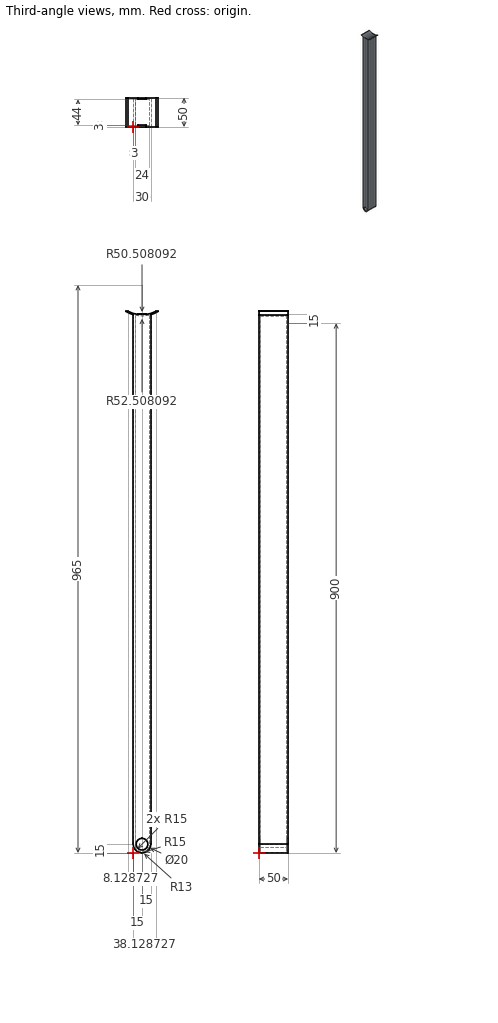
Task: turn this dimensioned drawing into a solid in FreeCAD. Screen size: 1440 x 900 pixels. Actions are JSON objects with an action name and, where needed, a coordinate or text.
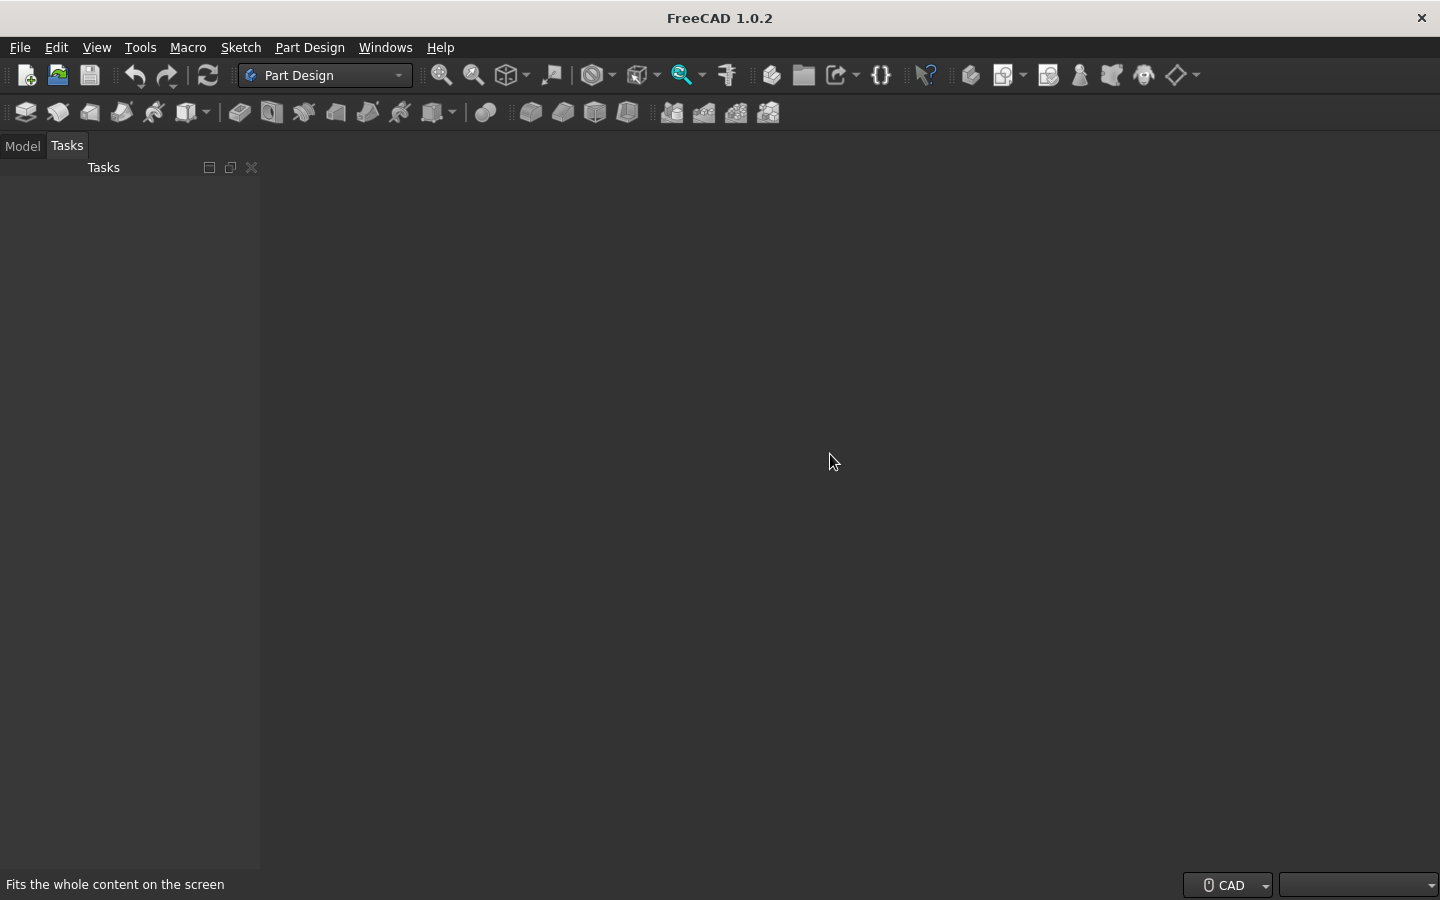
{"action": "left_click", "coordinate": [26, 76]}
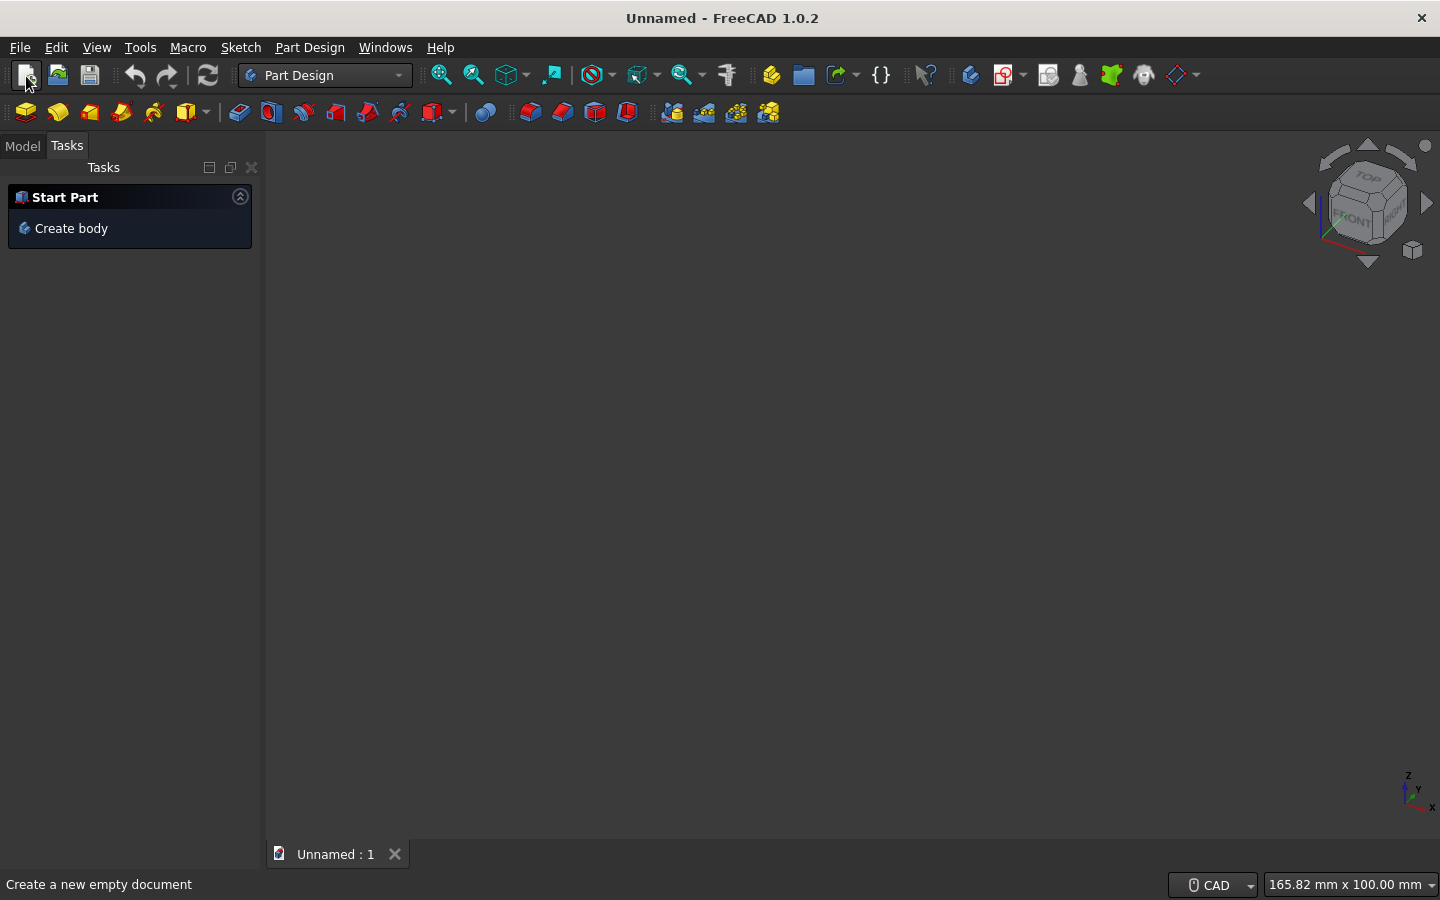
{"action": "left_click", "coordinate": [1004, 76]}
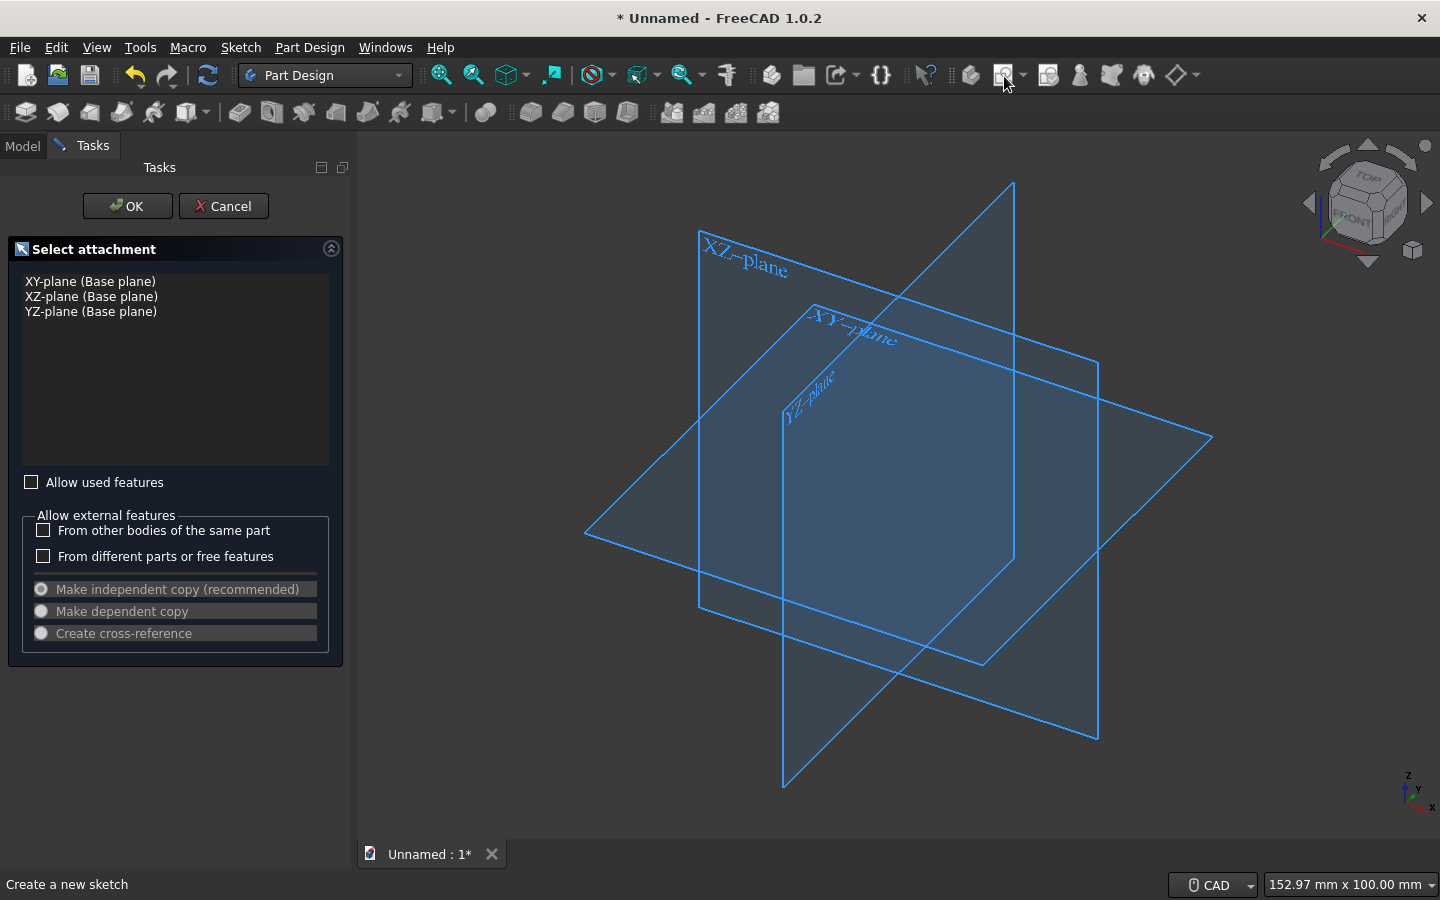
{"action": "left_click", "coordinate": [82, 282]}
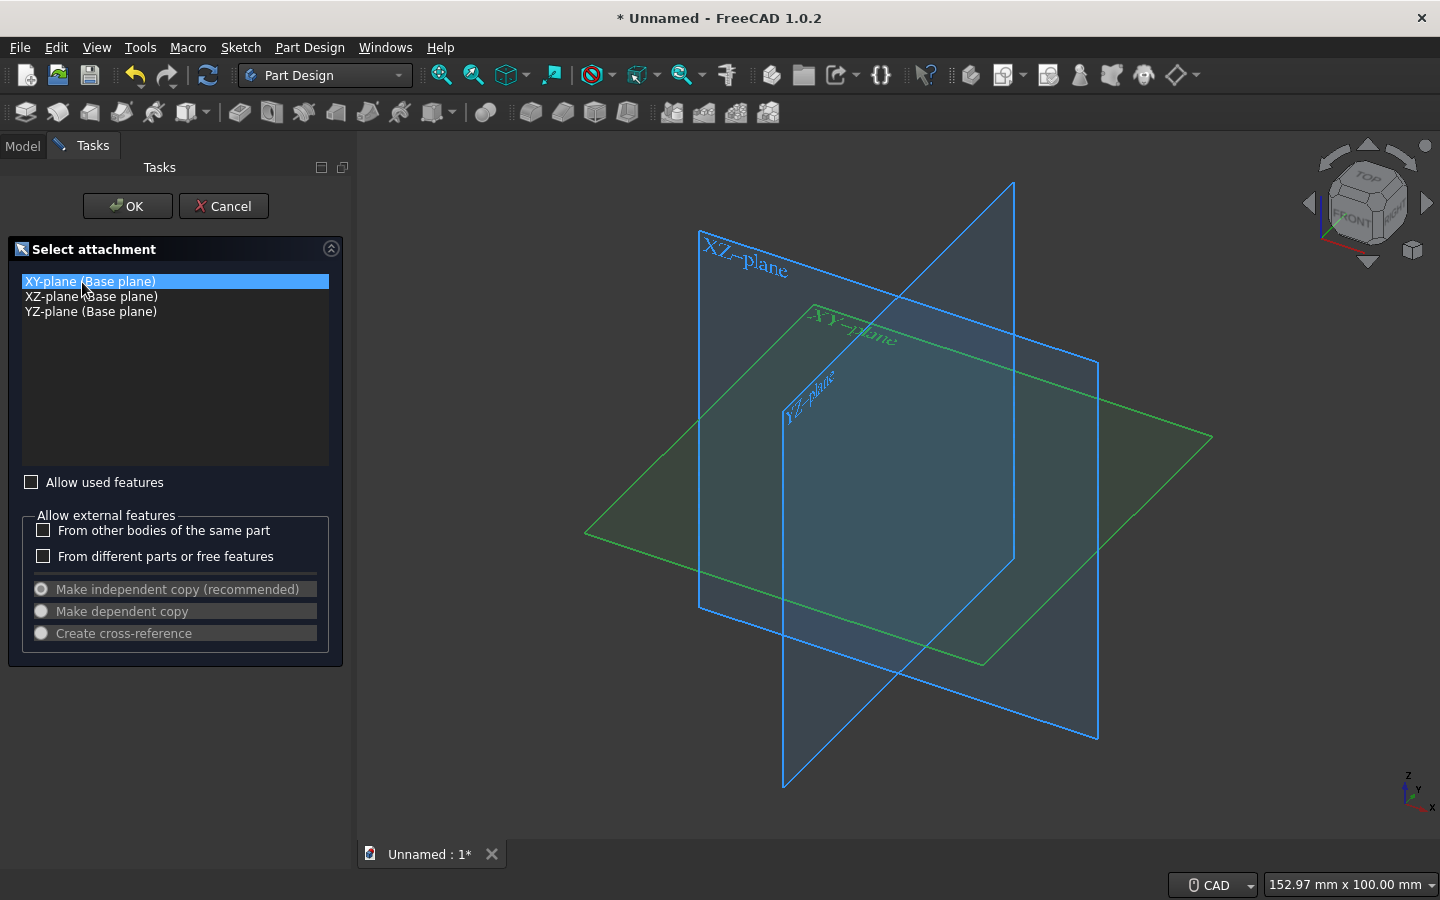
{"action": "left_click", "coordinate": [128, 206]}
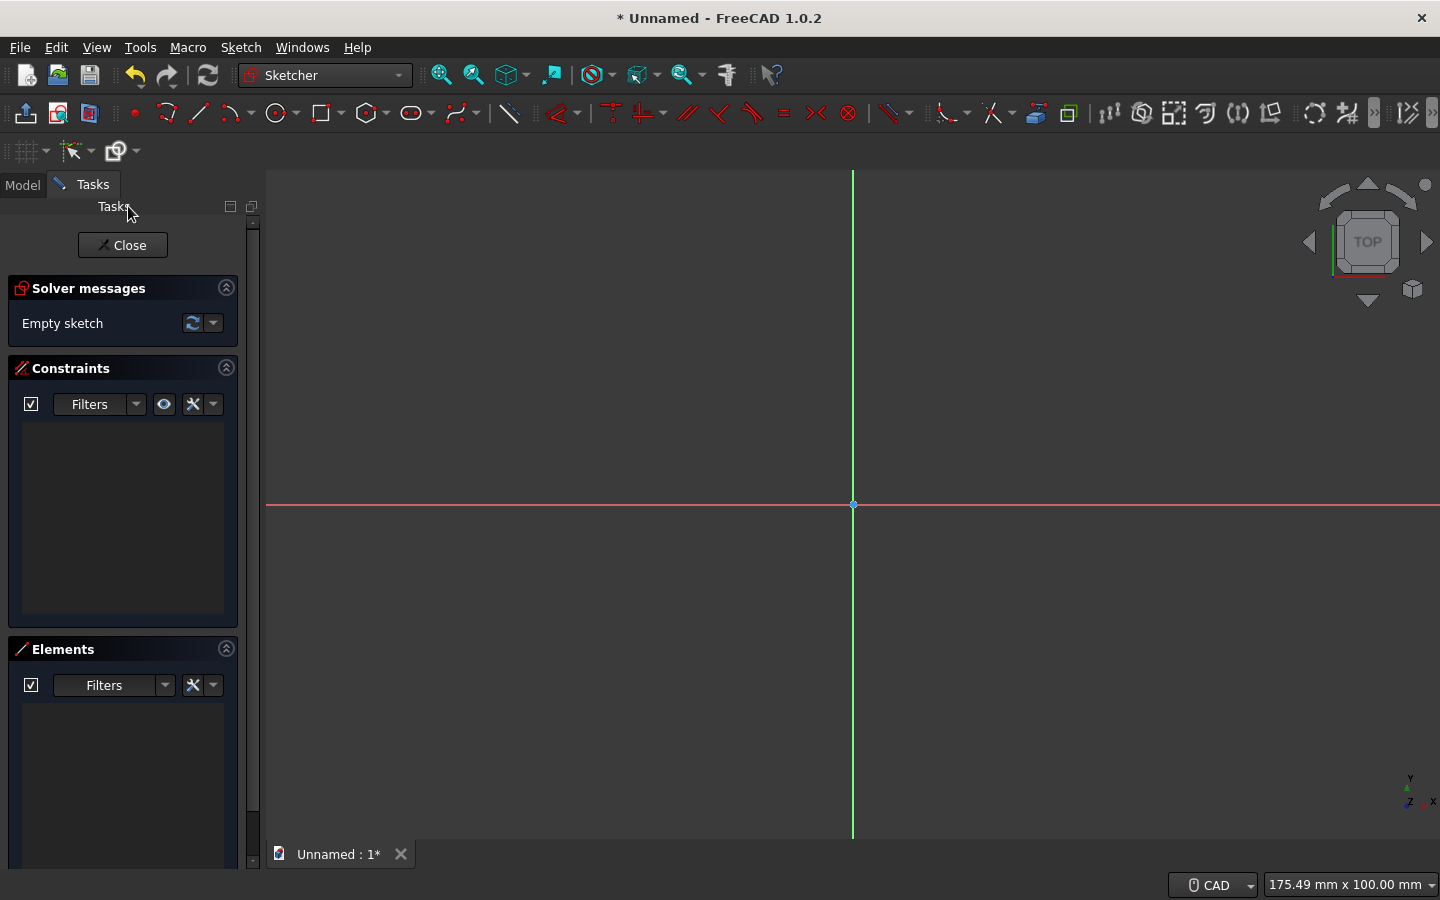
{"action": "scroll", "coordinate": [294, 811], "scroll_direction": "down", "scroll_amount": 1}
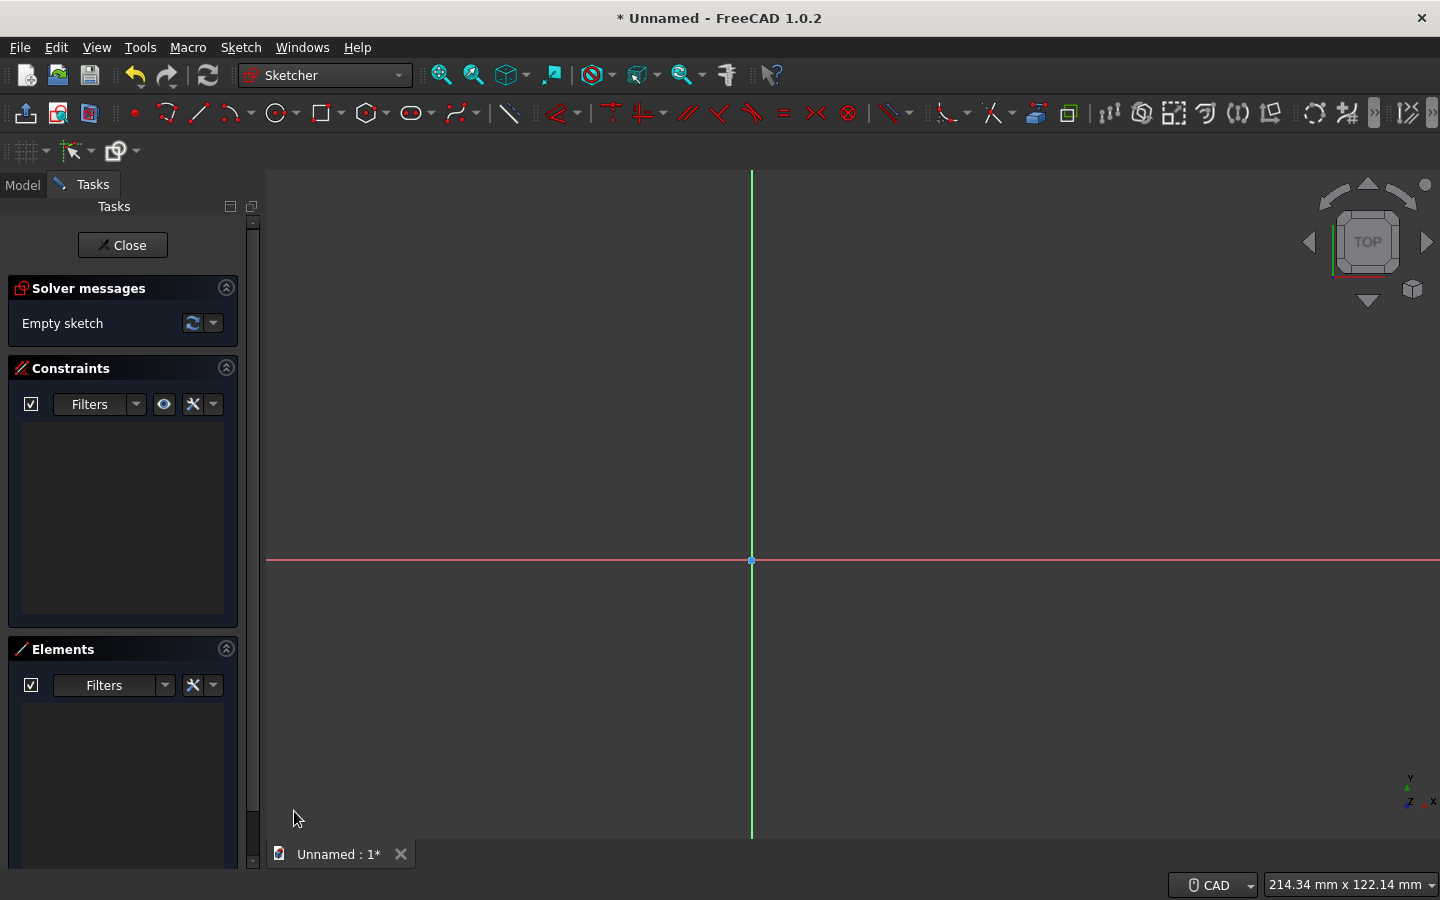
{"action": "scroll", "coordinate": [934, 258], "scroll_direction": "up", "scroll_amount": 2}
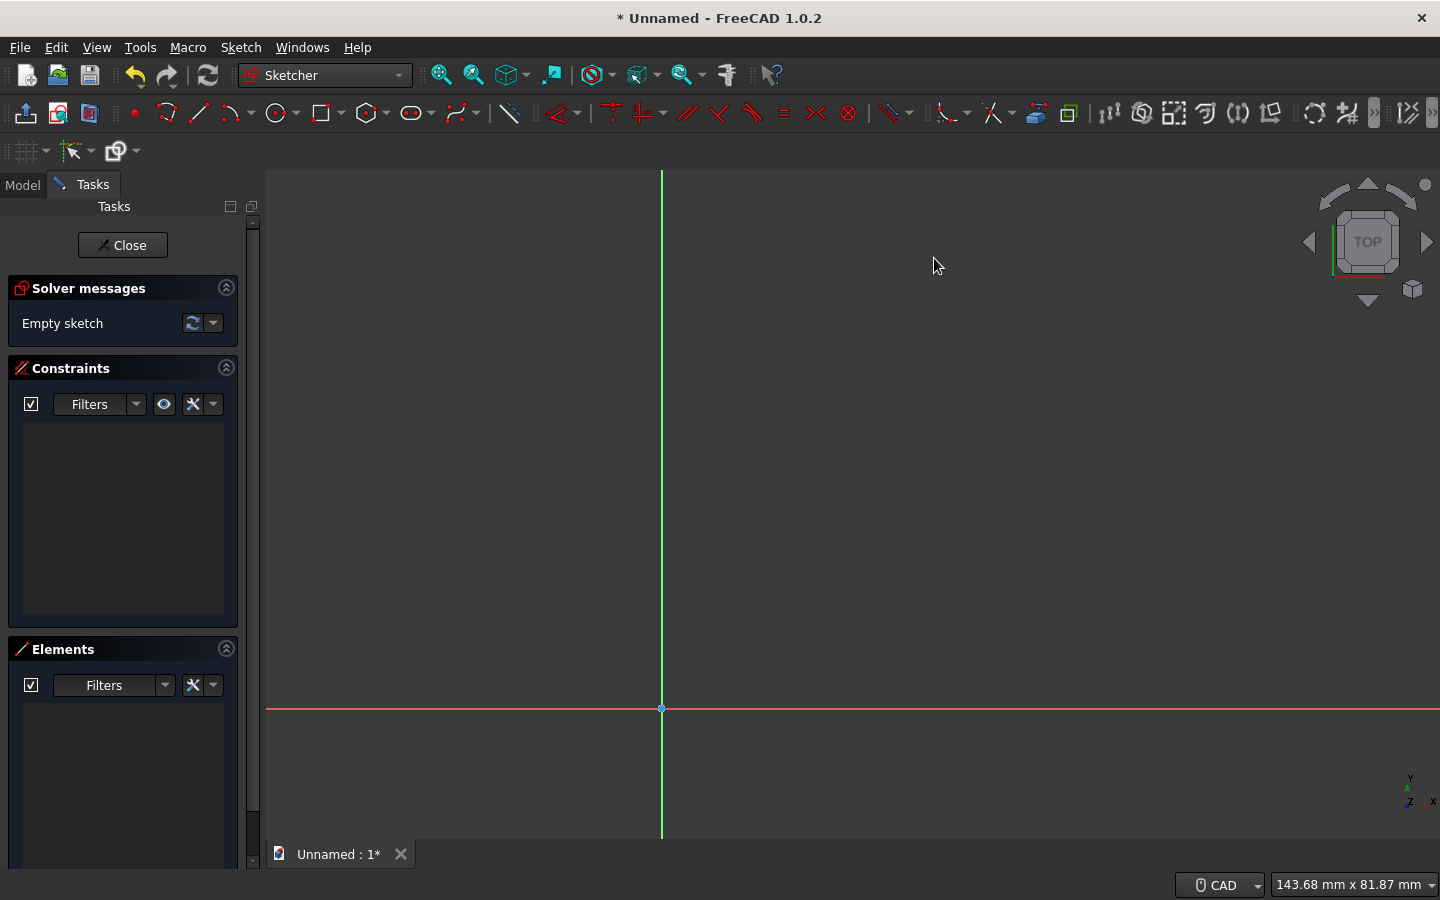
{"action": "left_click", "coordinate": [322, 114]}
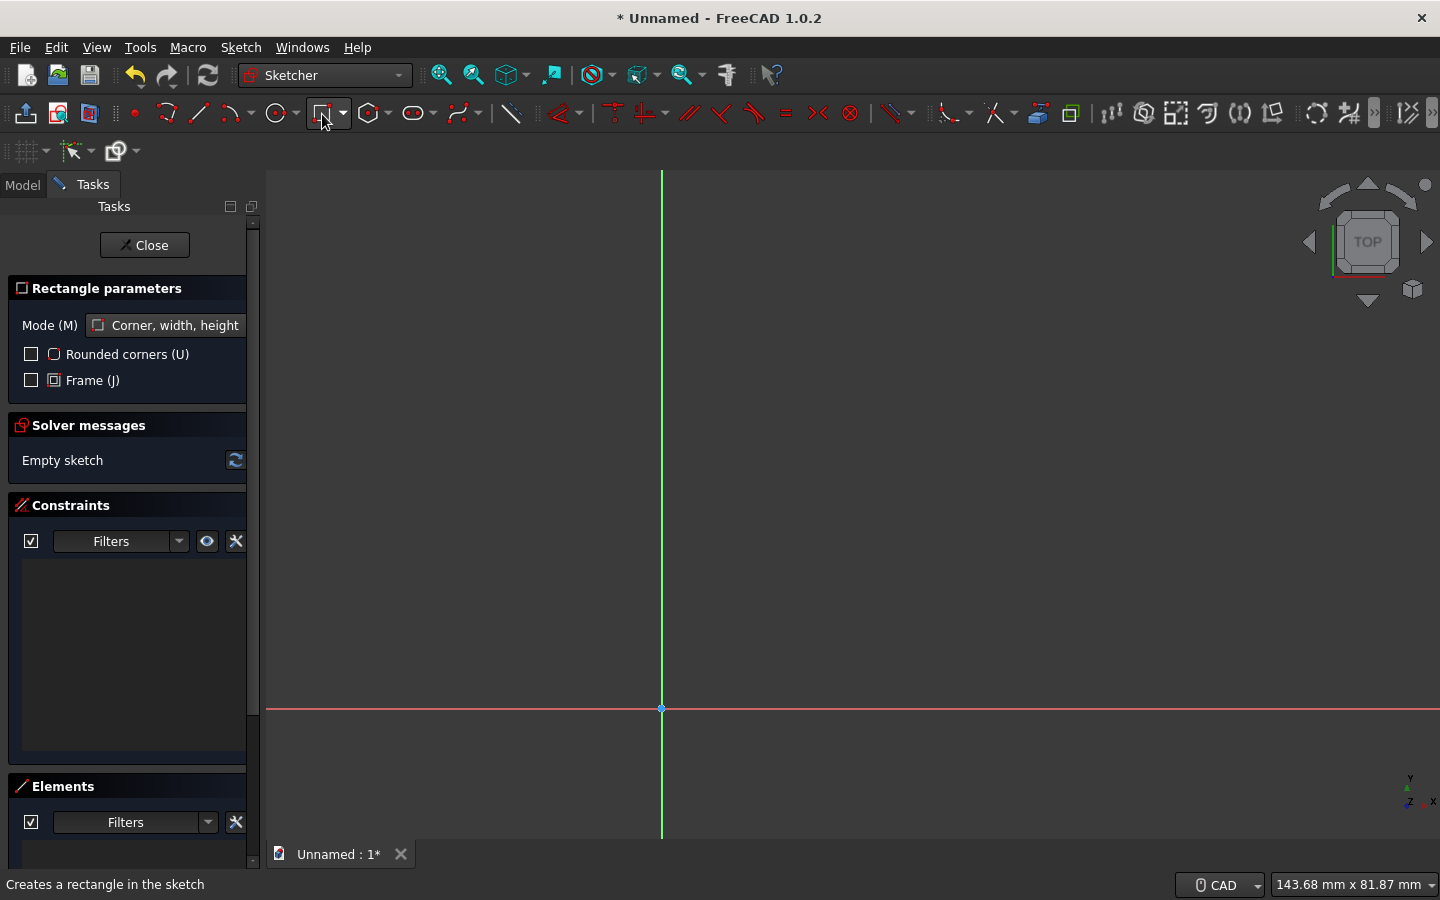
{"action": "left_click", "coordinate": [662, 709]}
{"action": "left_click", "coordinate": [907, 300]}